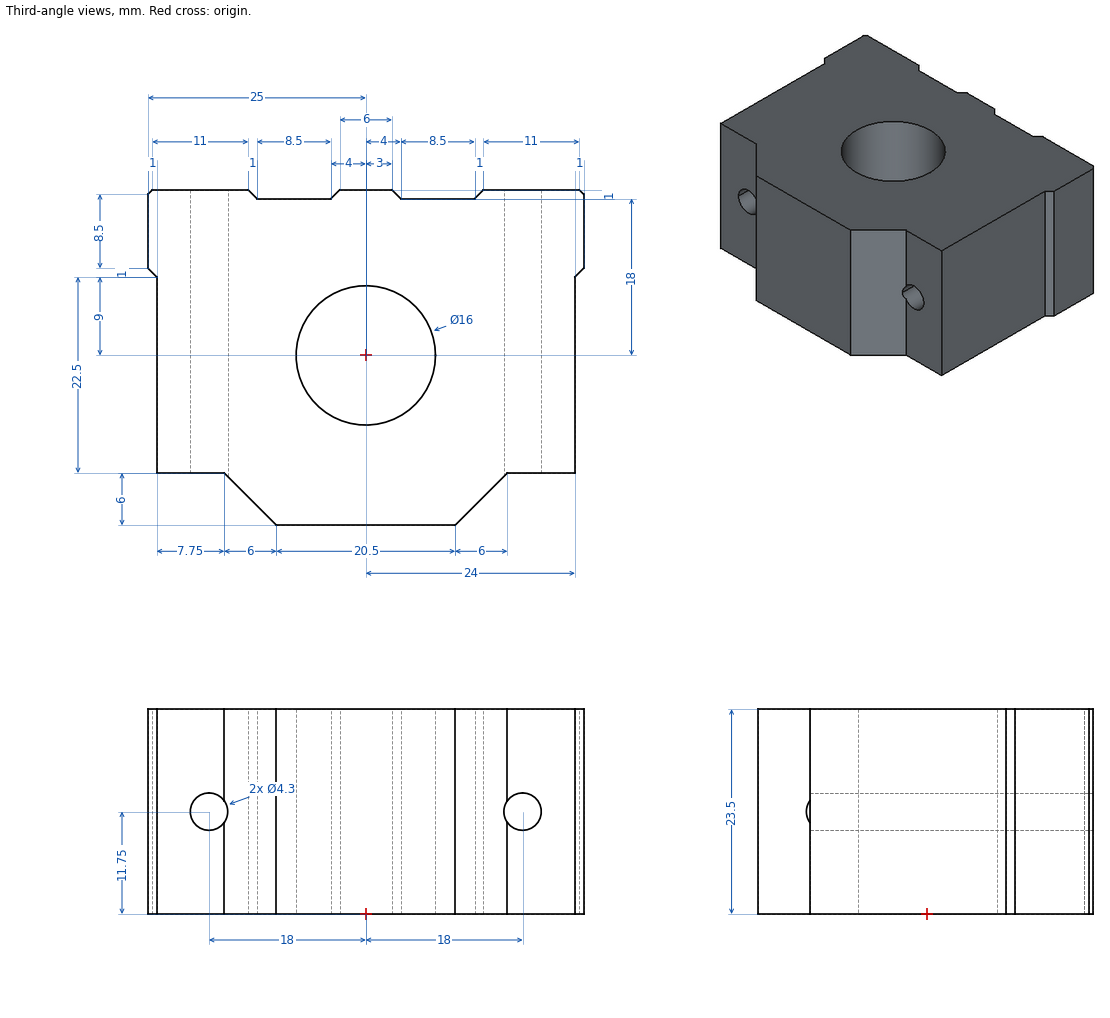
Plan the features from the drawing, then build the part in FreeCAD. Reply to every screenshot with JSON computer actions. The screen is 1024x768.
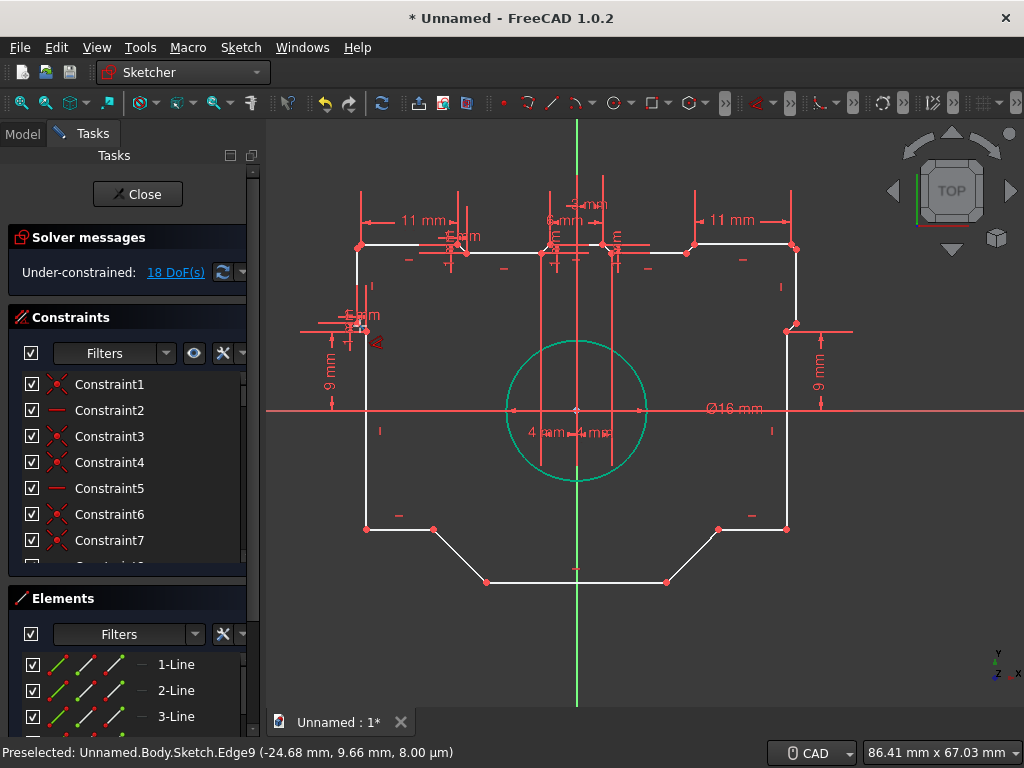
{"action": "left_click", "coordinate": [450, 546]}
{"action": "left_click", "coordinate": [460, 617]}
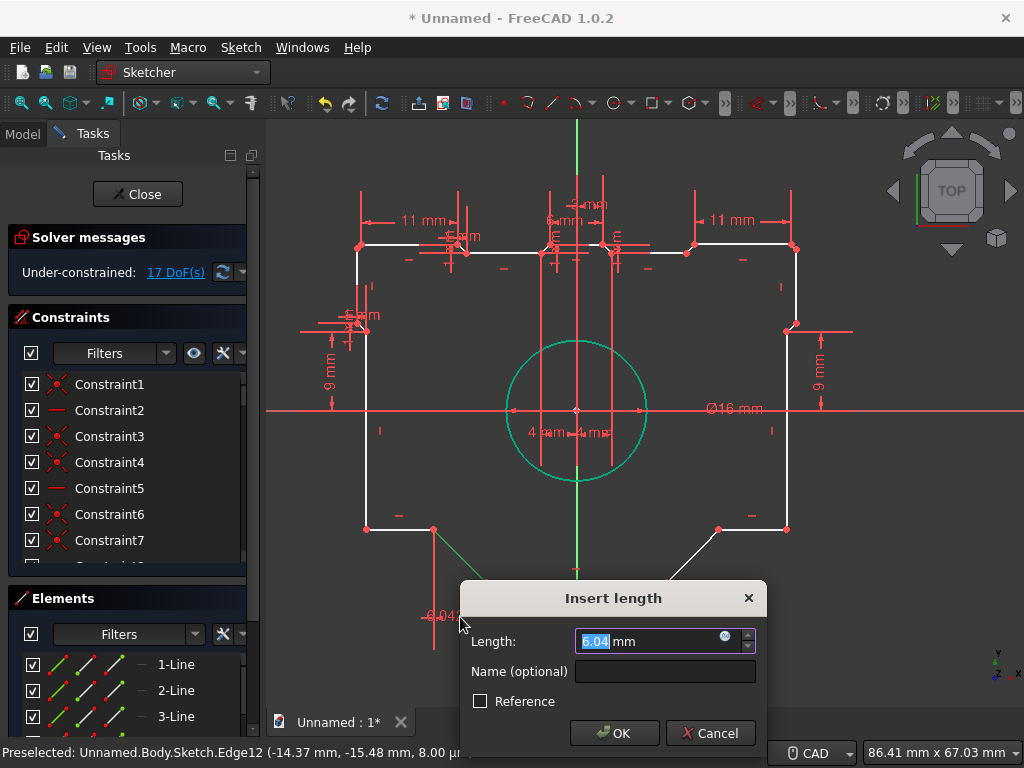
{"action": "type", "text": "6"}
{"action": "key", "text": "Return"}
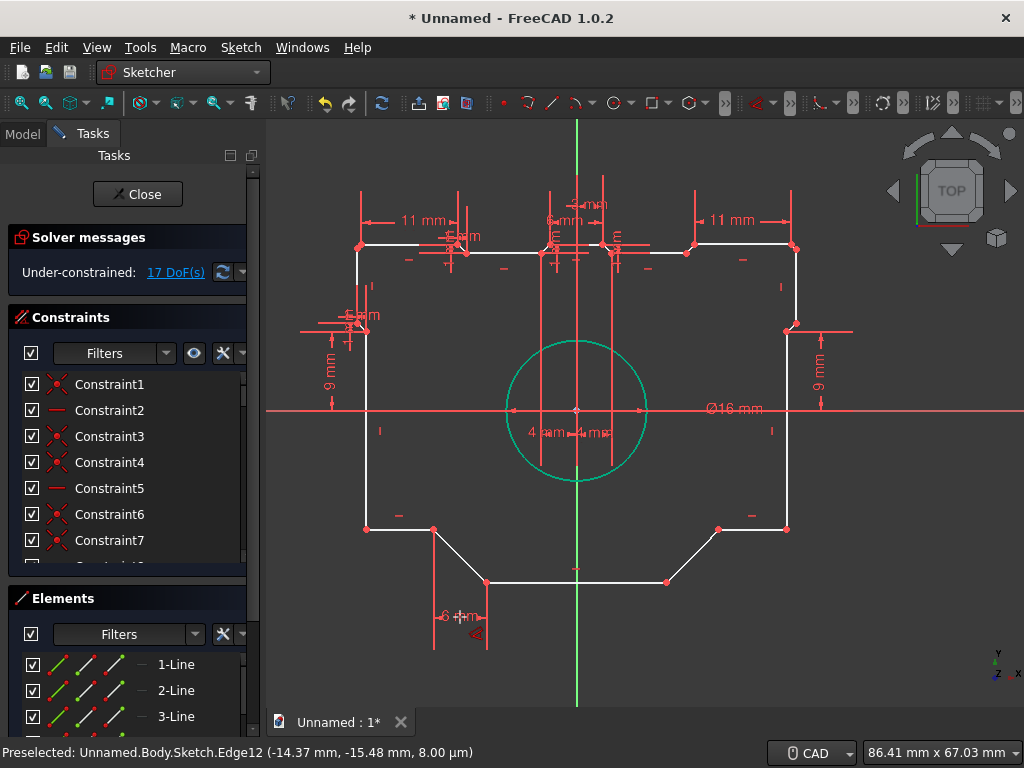
{"action": "left_click", "coordinate": [450, 546]}
{"action": "left_click", "coordinate": [400, 556]}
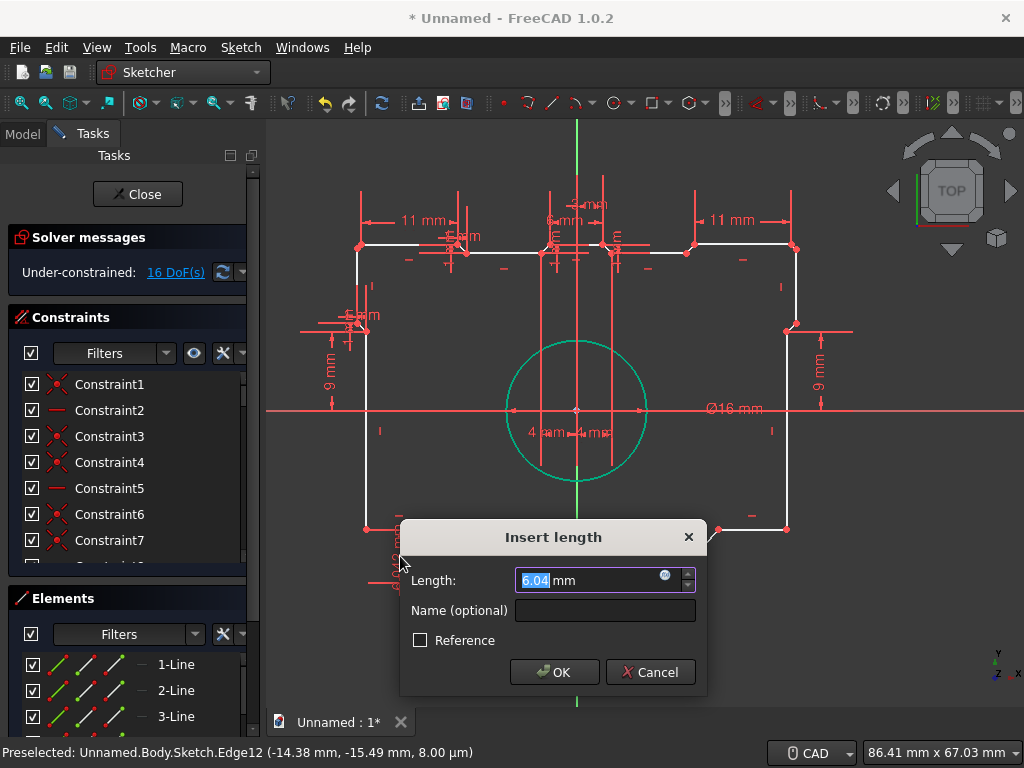
{"action": "type", "text": "6"}
{"action": "key", "text": "Return"}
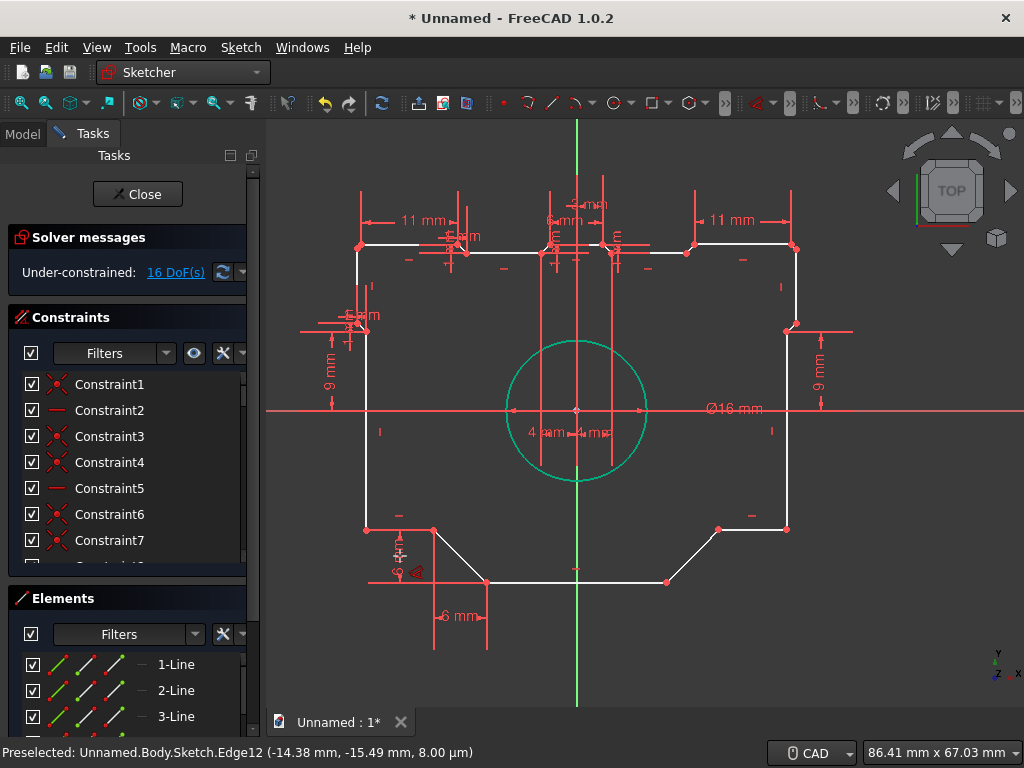
{"action": "left_click", "coordinate": [682, 567]}
{"action": "left_click", "coordinate": [693, 617]}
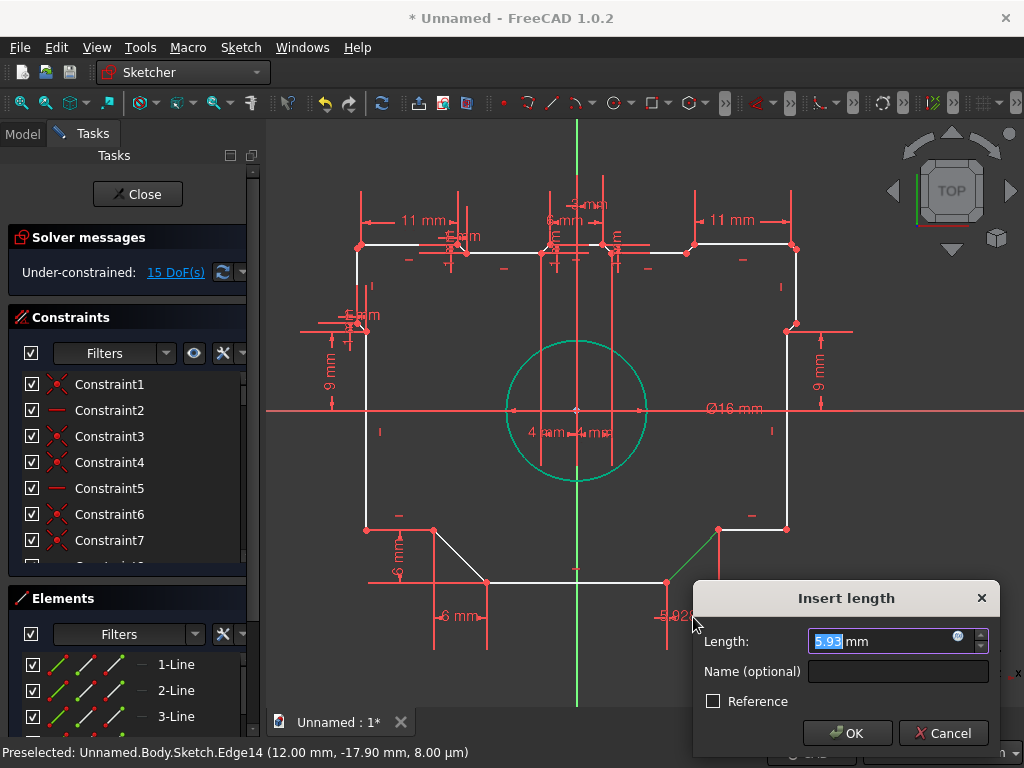
{"action": "type", "text": "6"}
{"action": "key", "text": "Return"}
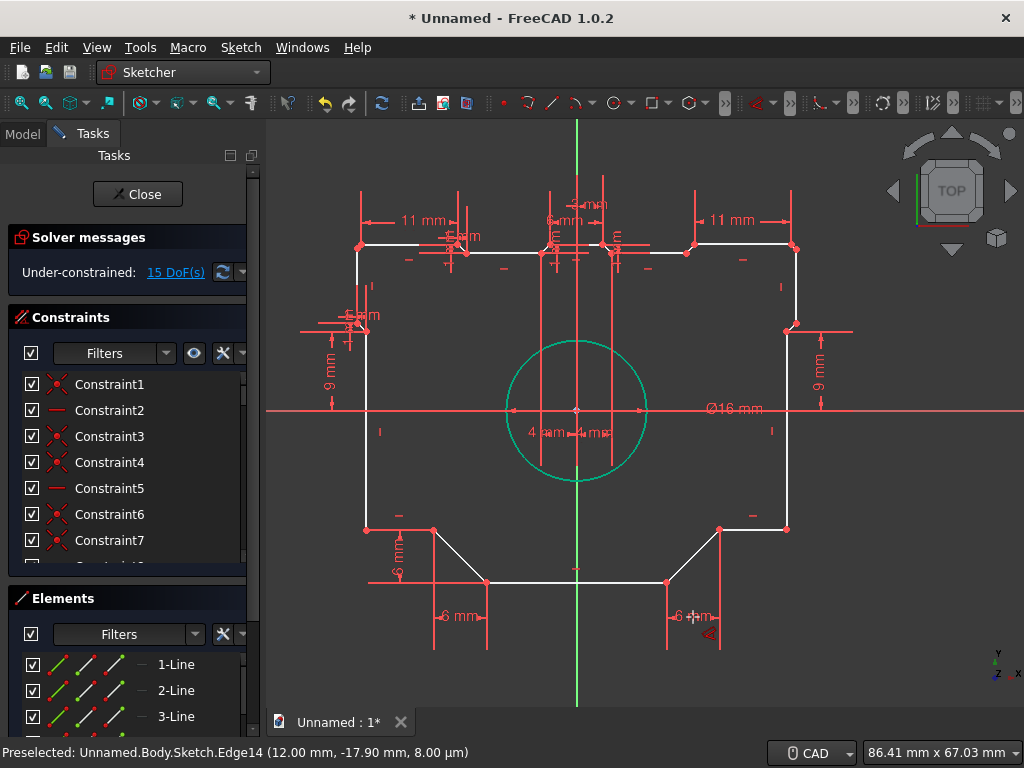
{"action": "left_click", "coordinate": [683, 567]}
{"action": "left_click", "coordinate": [754, 556]}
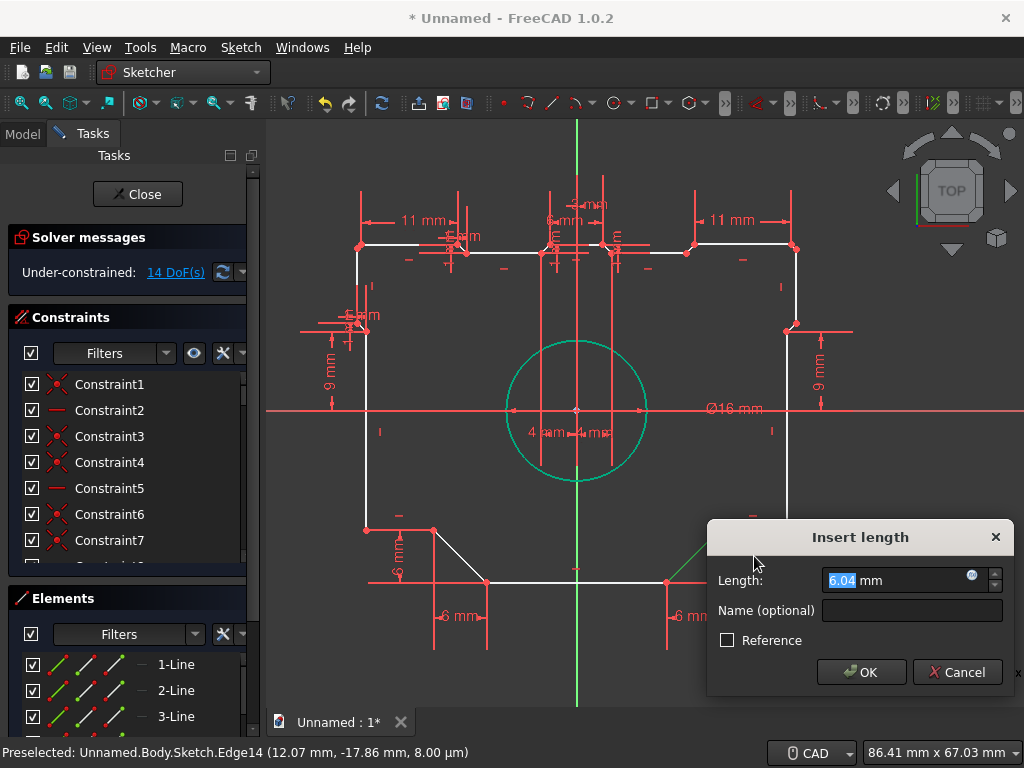
{"action": "type", "text": "6"}
{"action": "key", "text": "Return"}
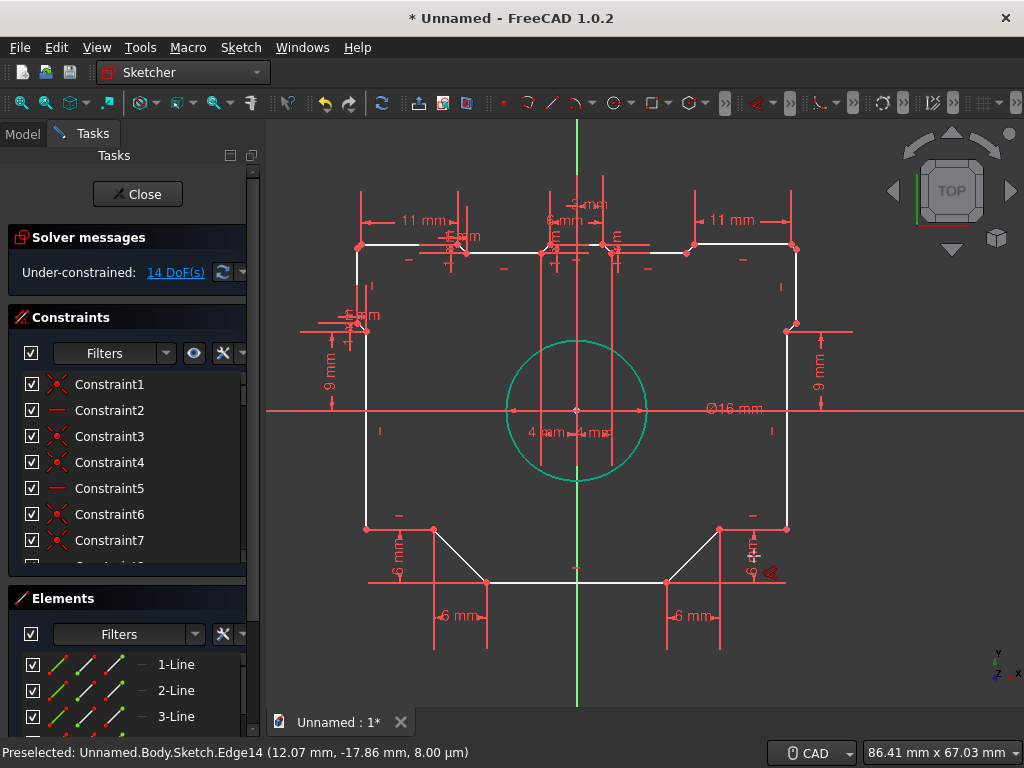
{"action": "scroll", "coordinate": [792, 328], "scroll_direction": "up", "scroll_amount": 8}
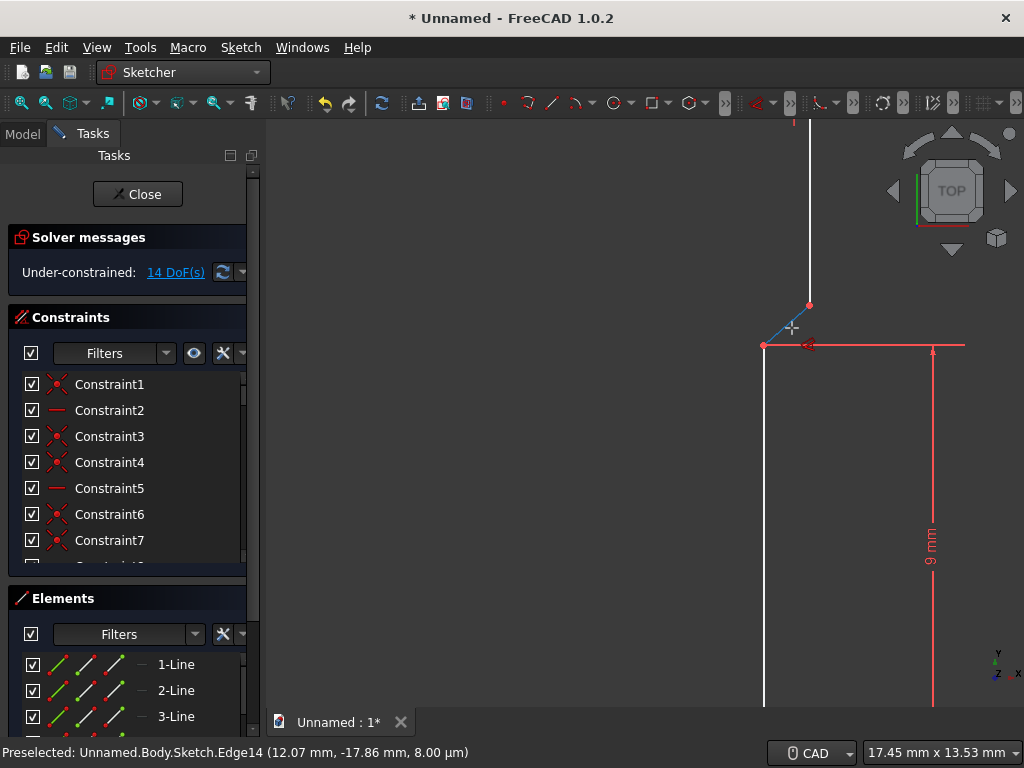
{"action": "left_click", "coordinate": [787, 325]}
{"action": "left_click", "coordinate": [787, 272]}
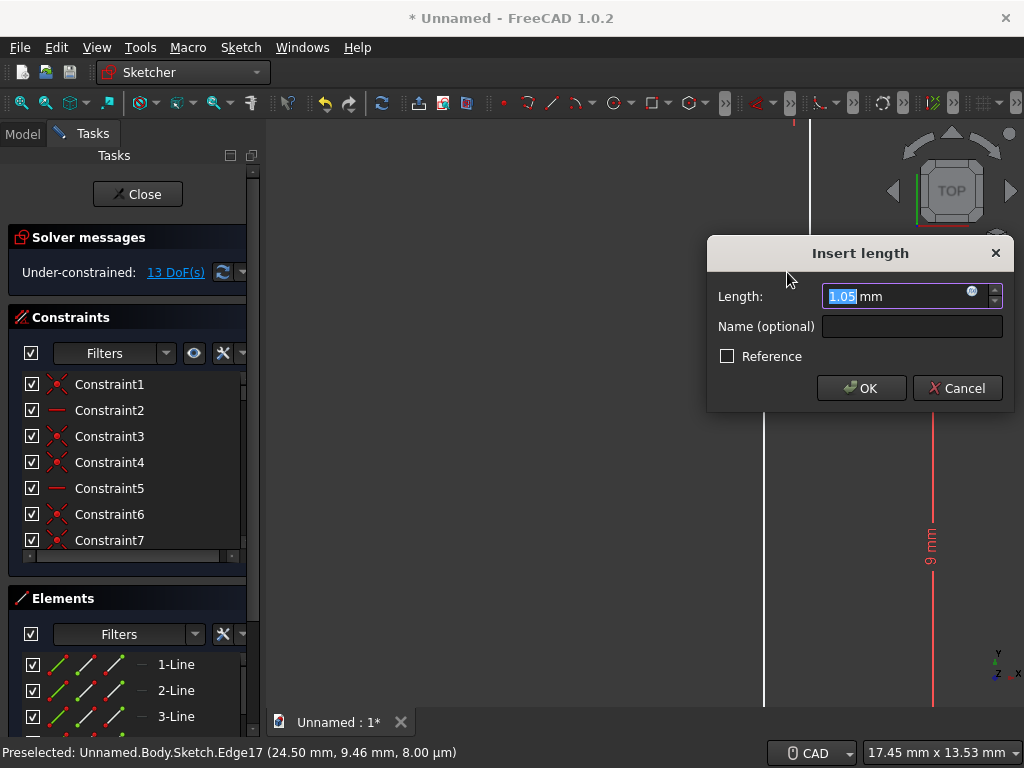
{"action": "type", "text": "1"}
{"action": "key", "text": "Return"}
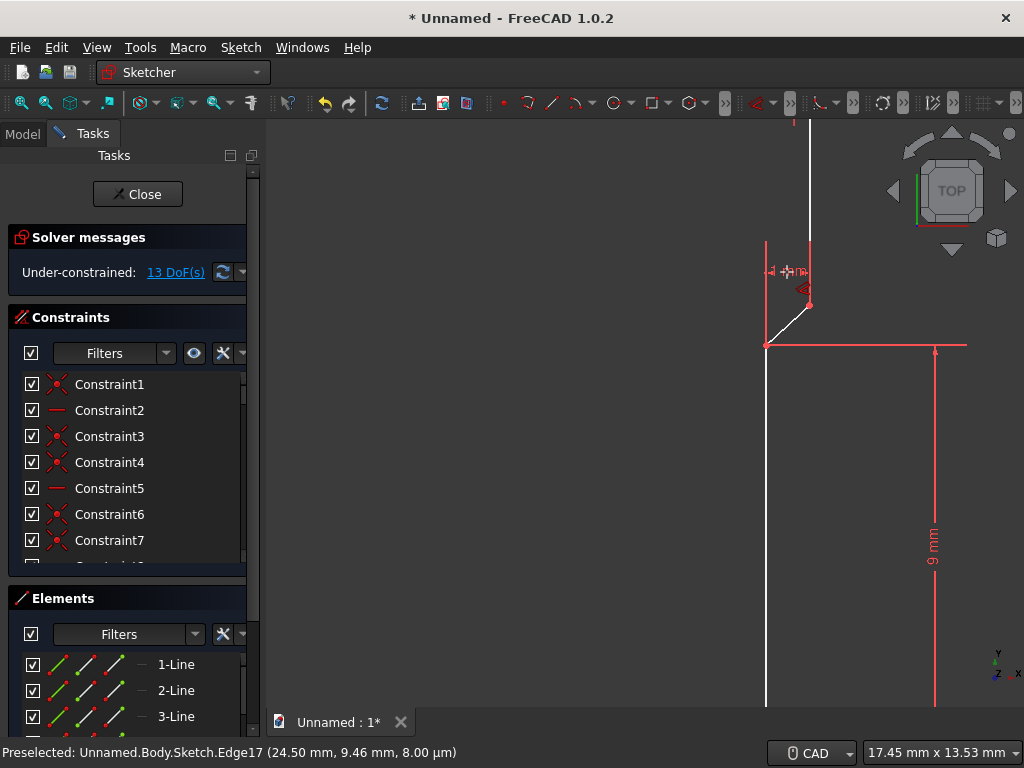
{"action": "left_click", "coordinate": [779, 333]}
{"action": "left_click", "coordinate": [844, 325]}